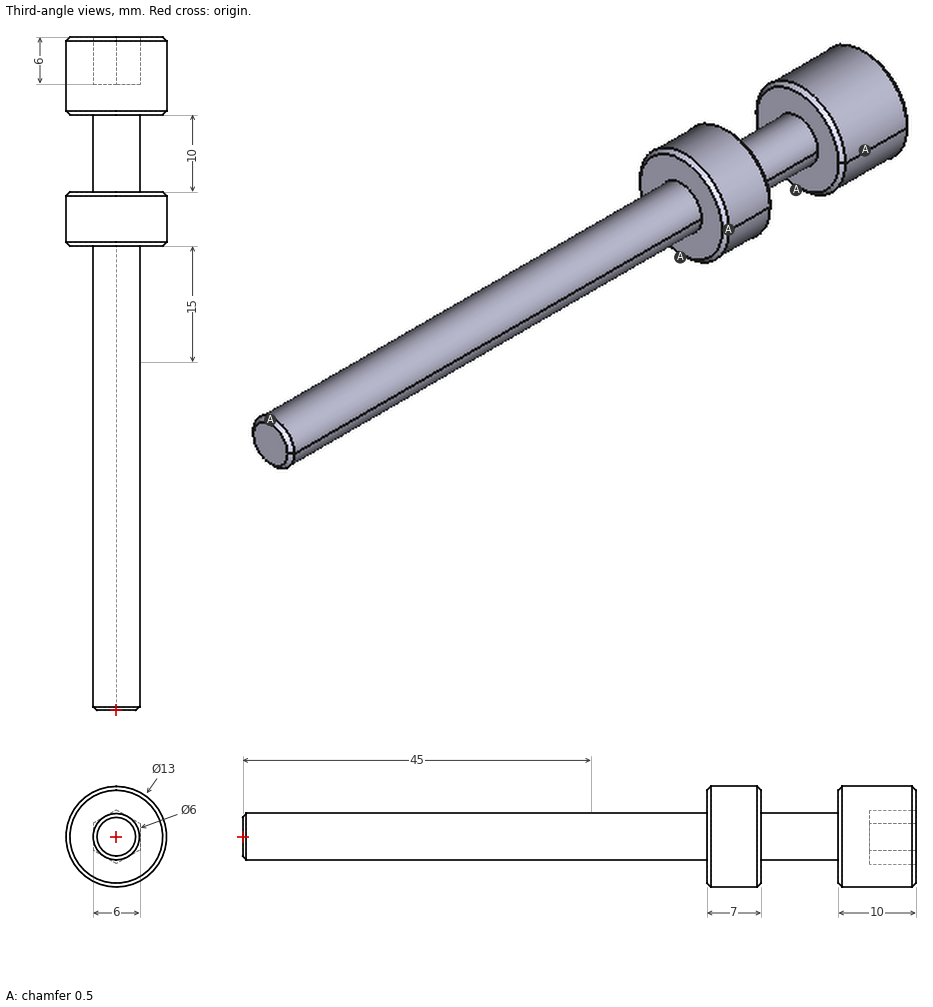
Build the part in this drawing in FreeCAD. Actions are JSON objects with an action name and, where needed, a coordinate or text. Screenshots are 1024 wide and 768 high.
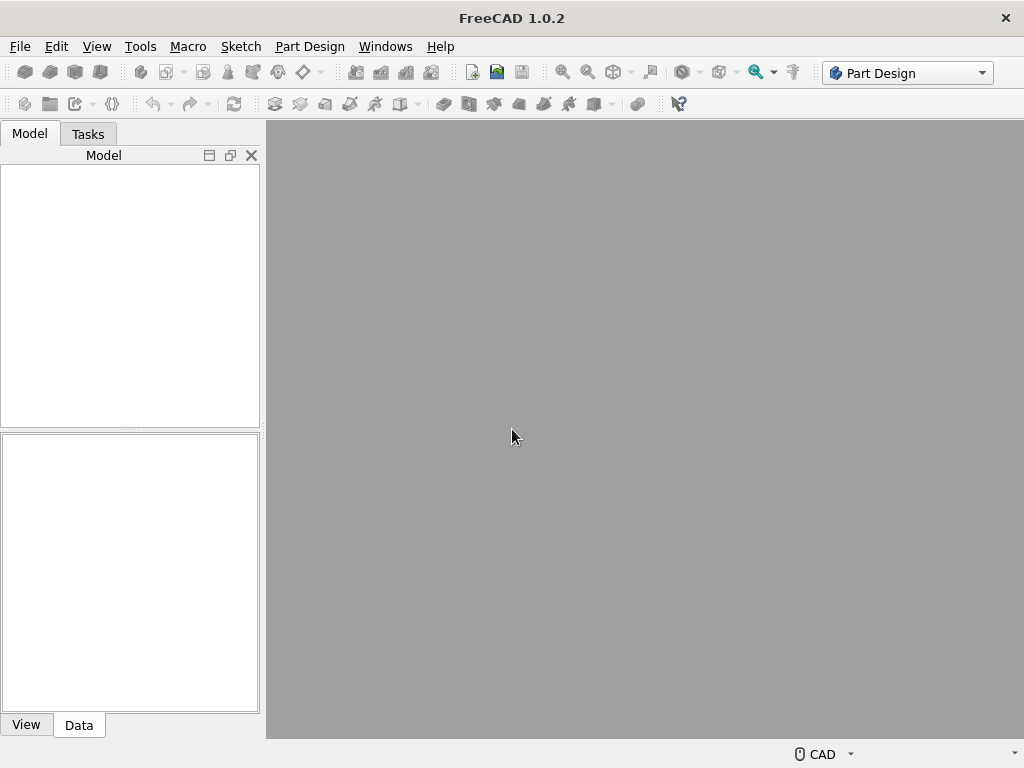
{"action": "key", "text": "ctrl+n"}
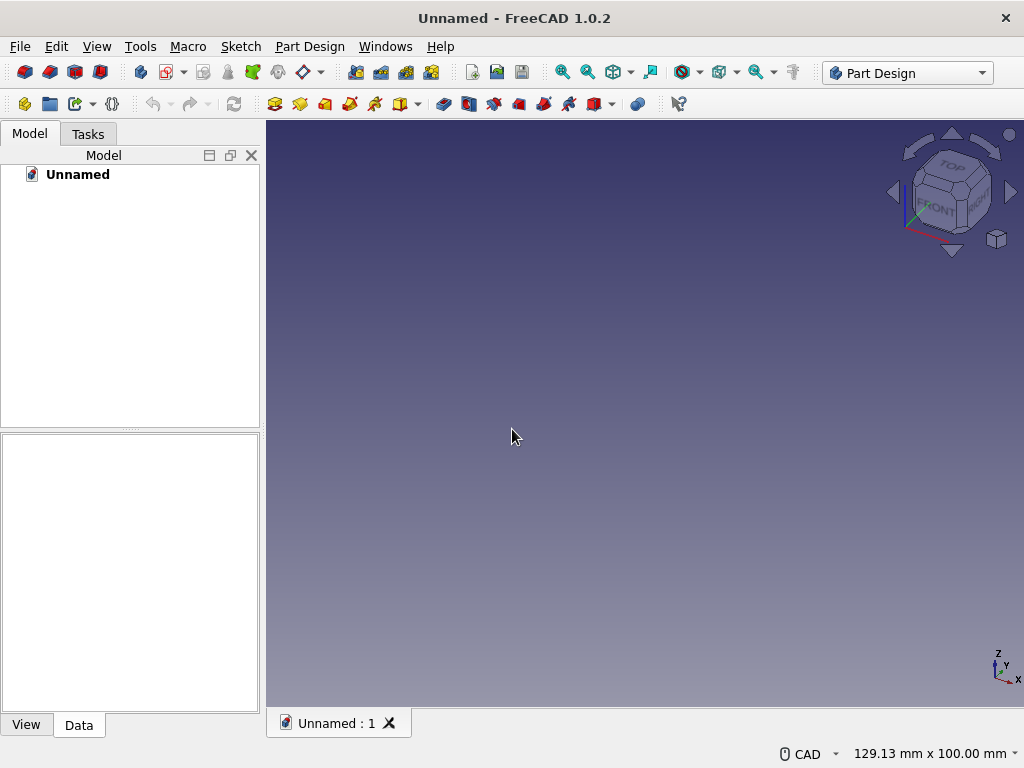
{"action": "left_click", "coordinate": [166, 72]}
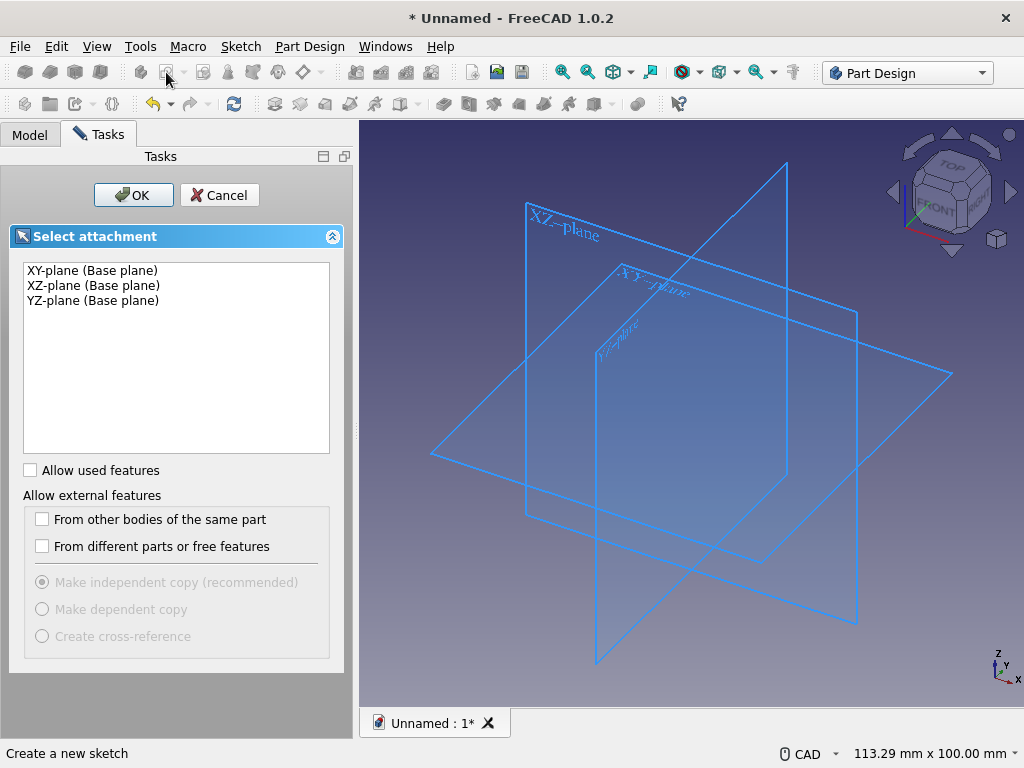
{"action": "left_click", "coordinate": [84, 286]}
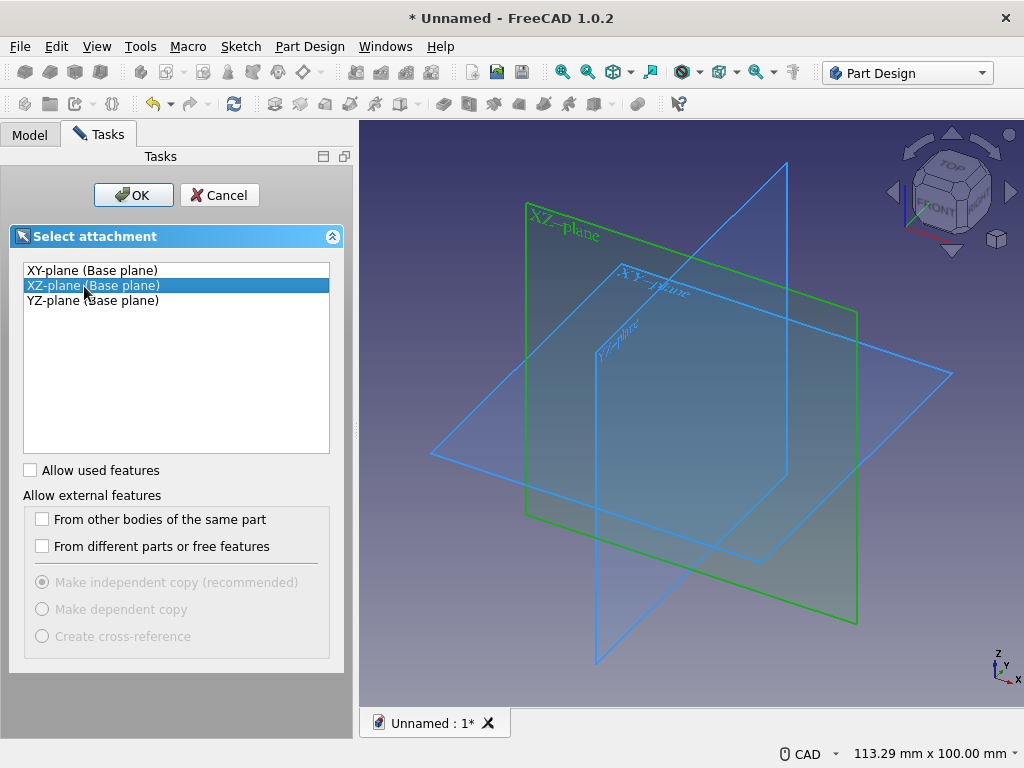
{"action": "left_click", "coordinate": [134, 195]}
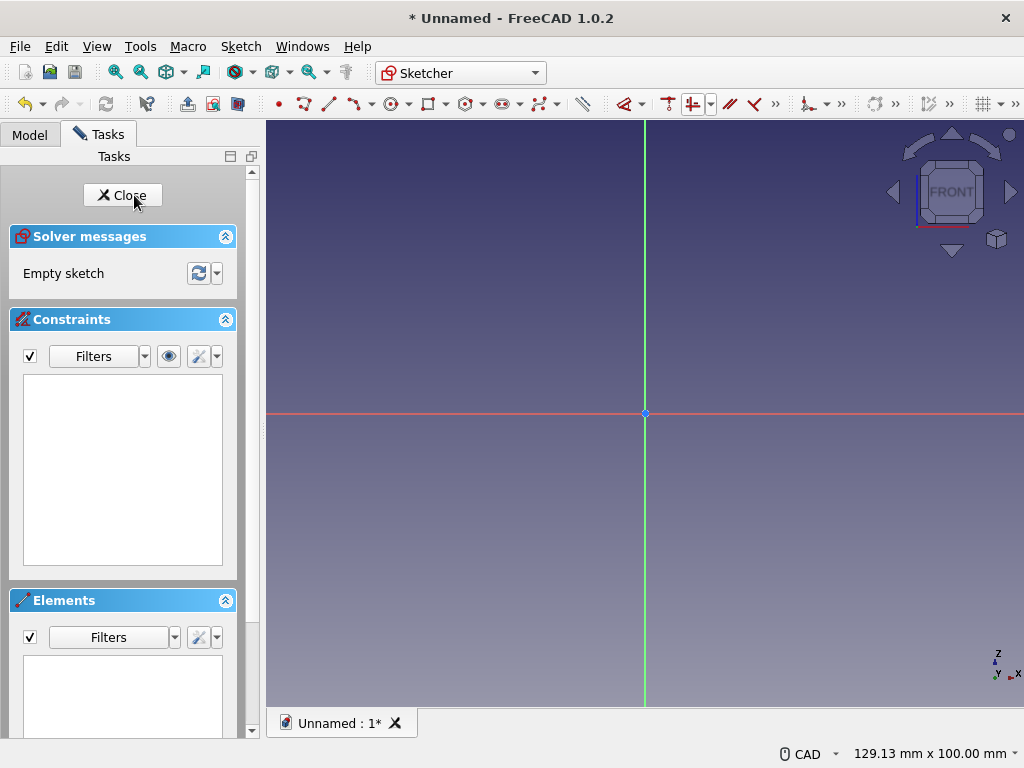
{"action": "scroll", "coordinate": [652, 414], "scroll_direction": "up", "scroll_amount": 12}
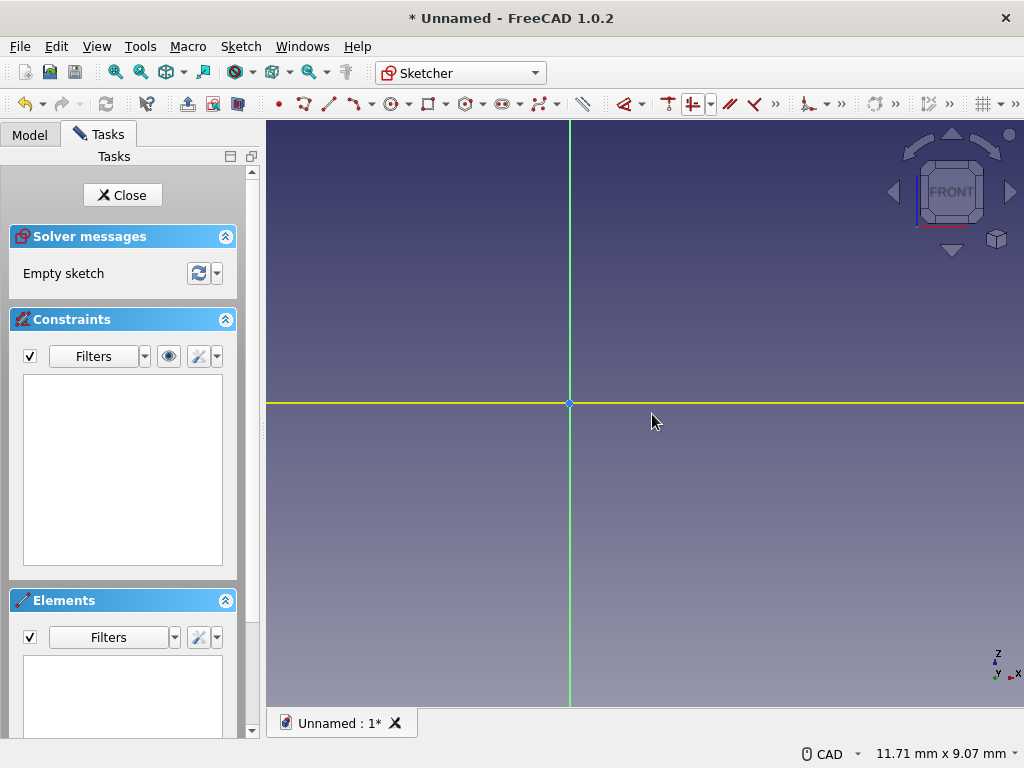
{"action": "left_click", "coordinate": [390, 104]}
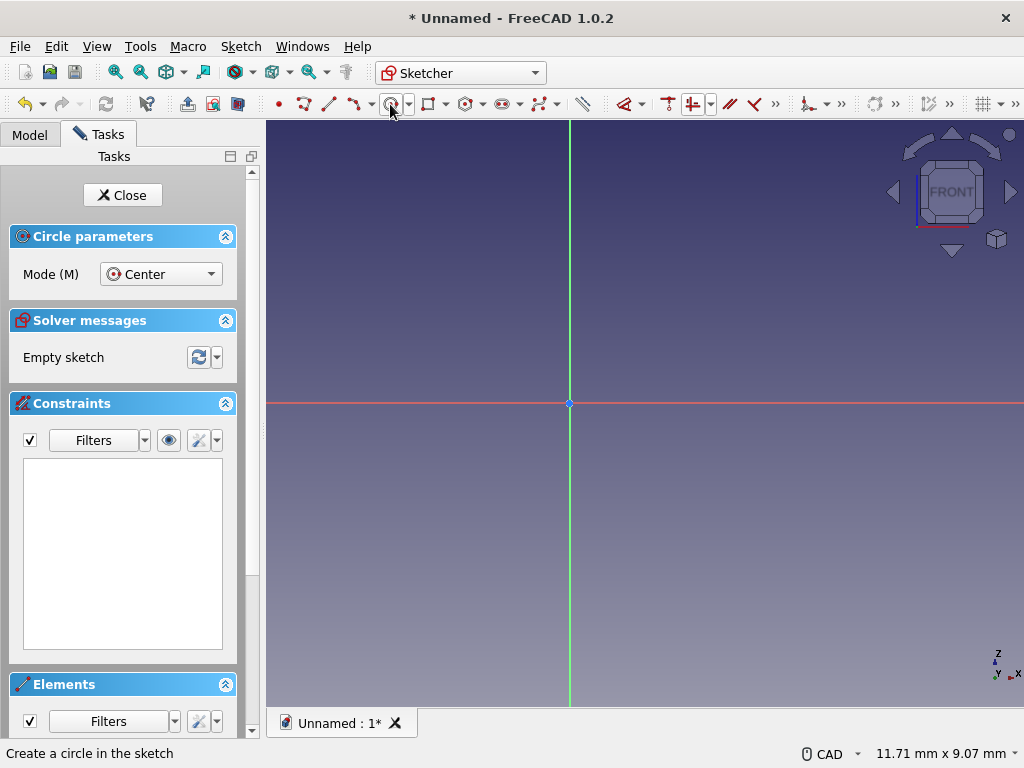
{"action": "left_click", "coordinate": [570, 403]}
{"action": "left_click", "coordinate": [707, 266]}
{"action": "key", "text": "Escape"}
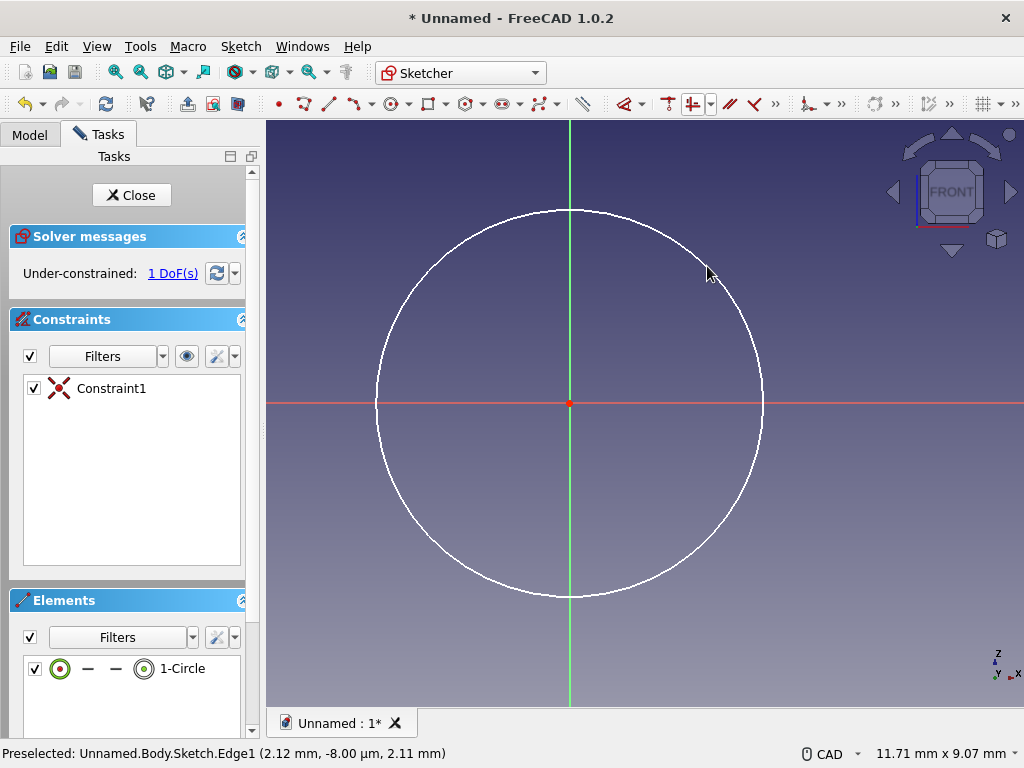
{"action": "left_click", "coordinate": [706, 266]}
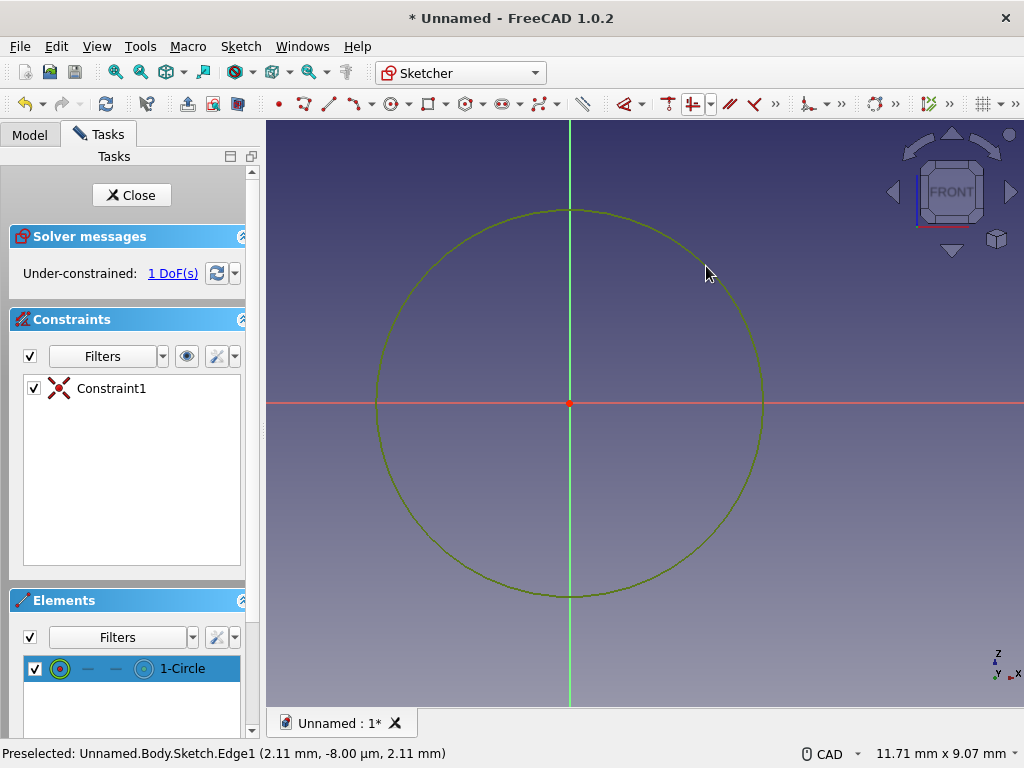
{"action": "key", "text": "k o"}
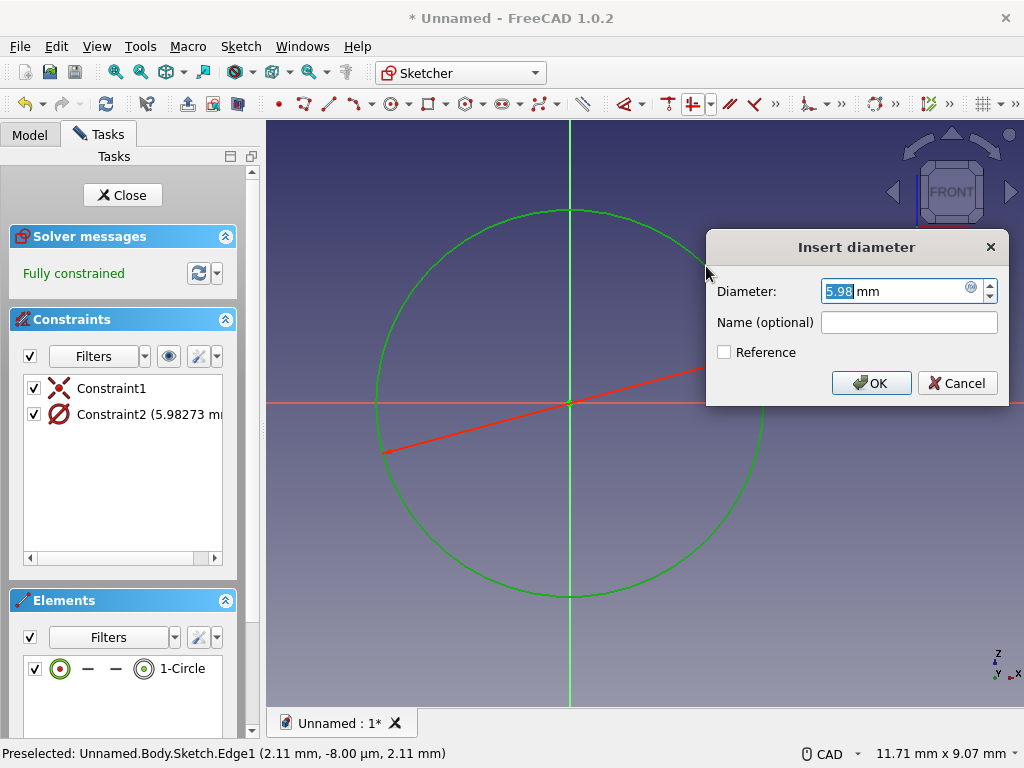
{"action": "type", "text": "6"}
{"action": "key", "text": "Return"}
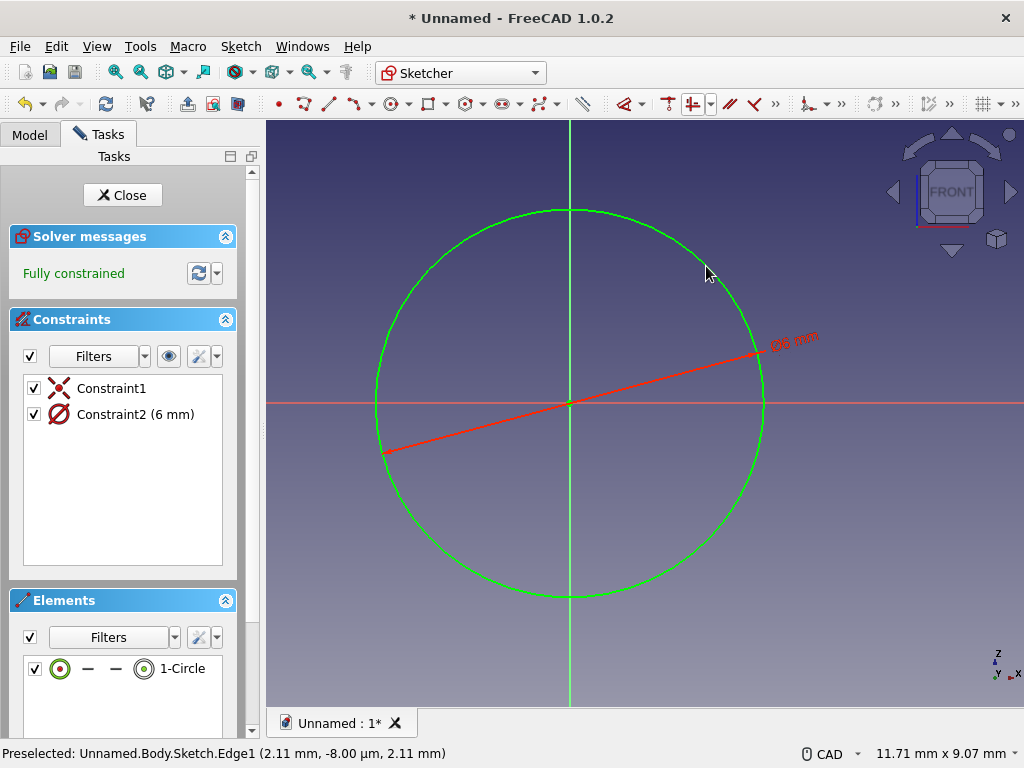
{"action": "left_click", "coordinate": [123, 195]}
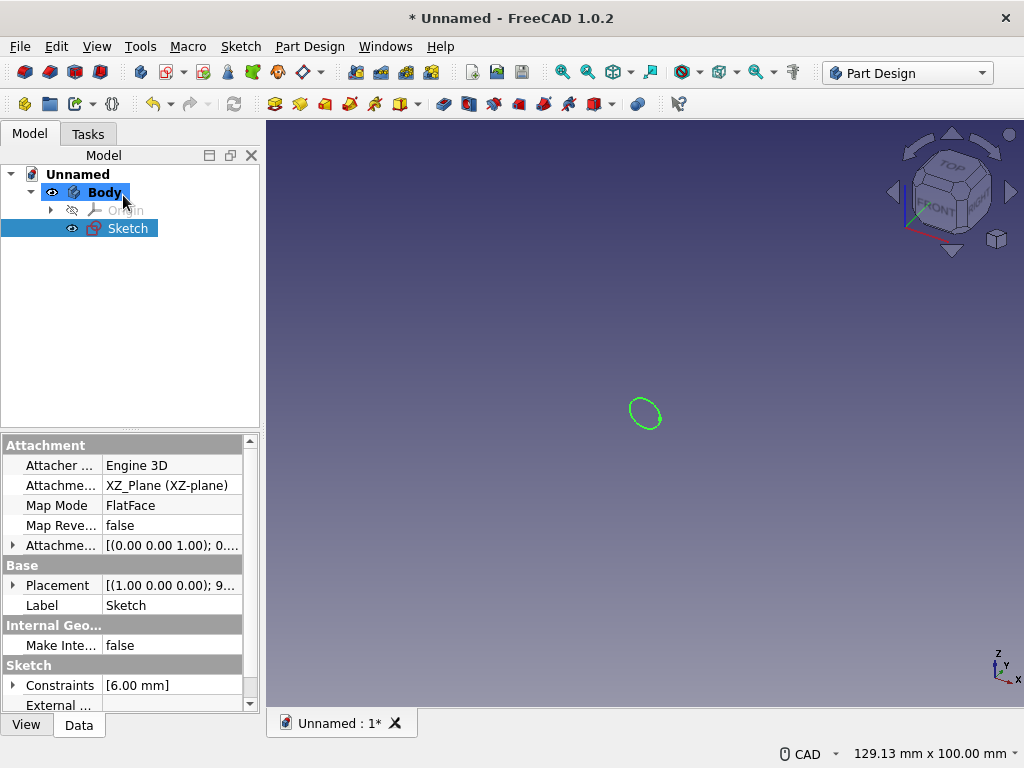
{"action": "left_click", "coordinate": [275, 104]}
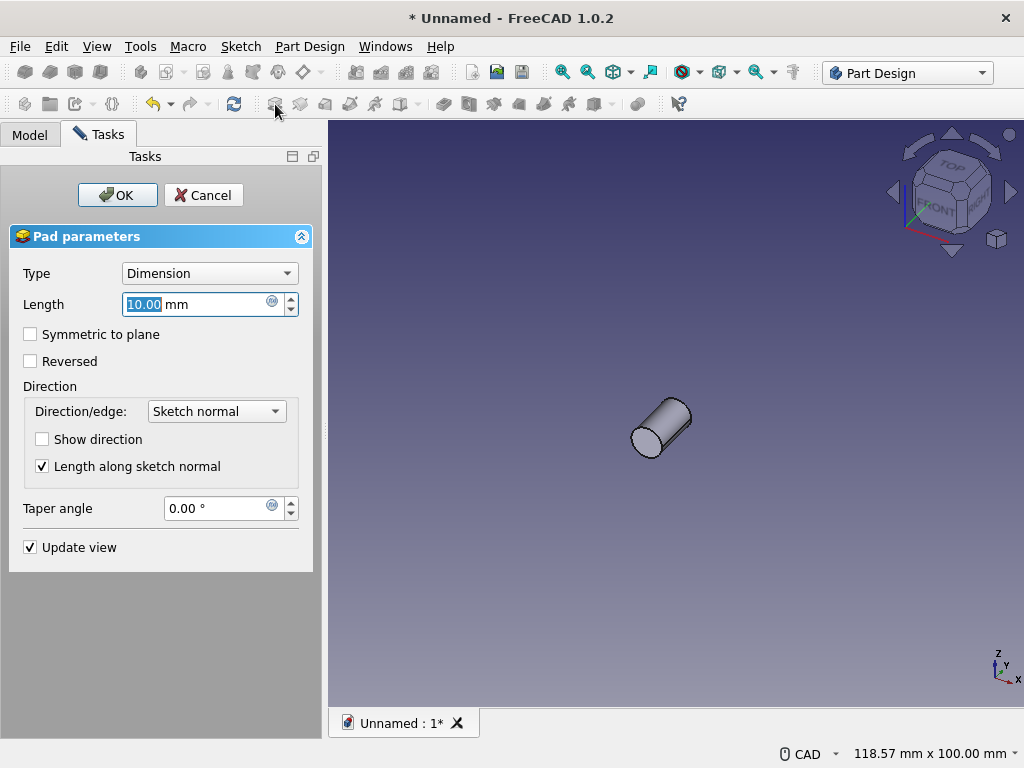
{"action": "type", "text": "45"}
{"action": "key", "text": "Tab"}